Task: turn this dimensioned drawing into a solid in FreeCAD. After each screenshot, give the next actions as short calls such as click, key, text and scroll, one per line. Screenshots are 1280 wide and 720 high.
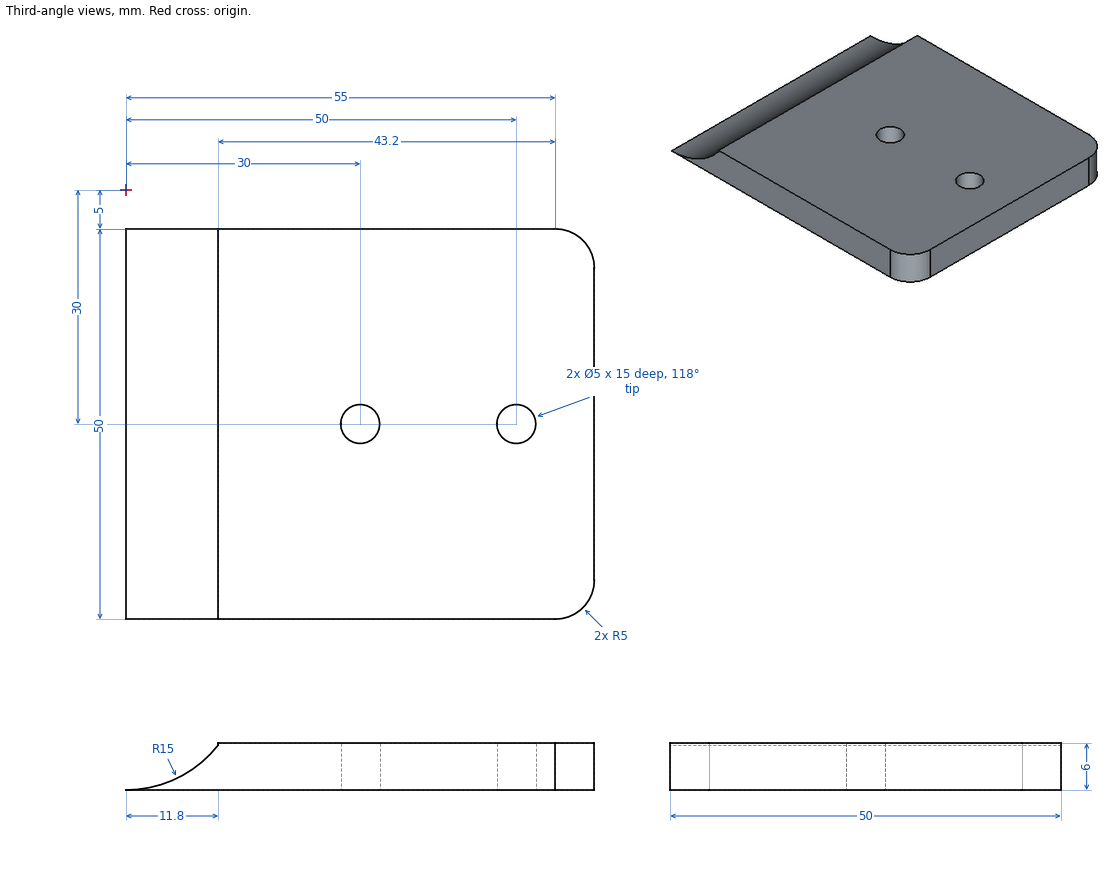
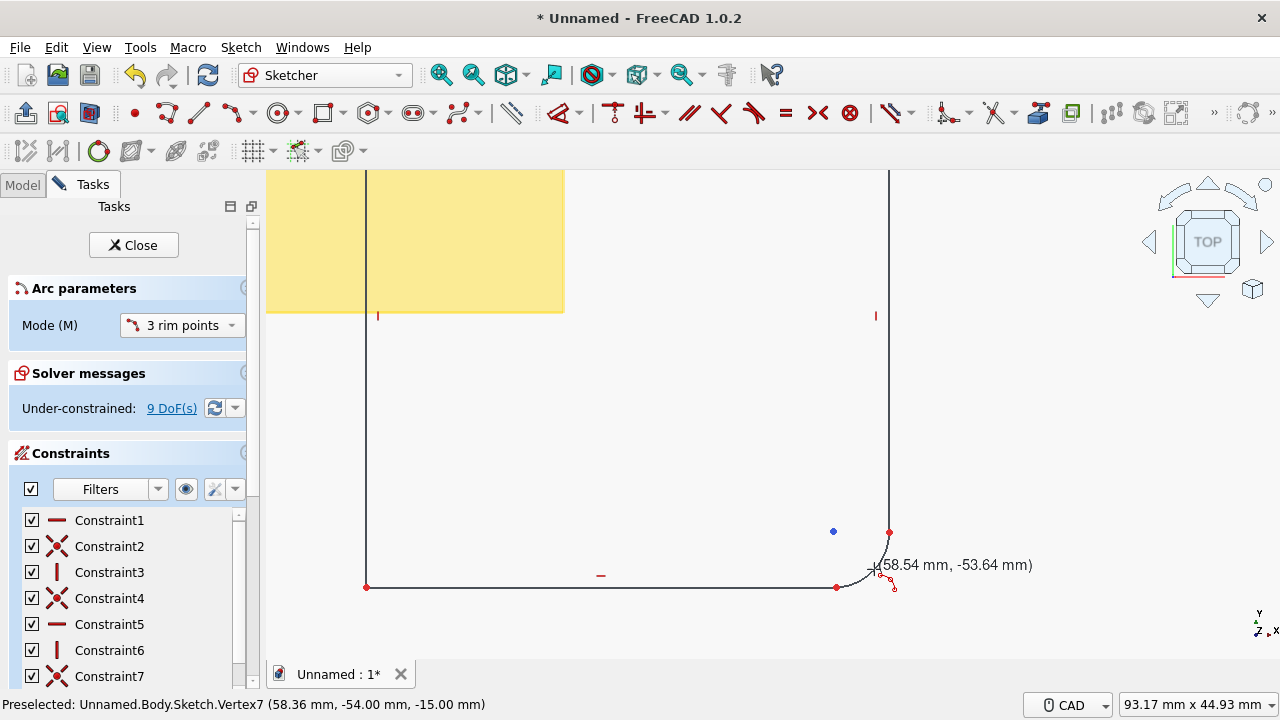
scroll(876, 571, down, 3)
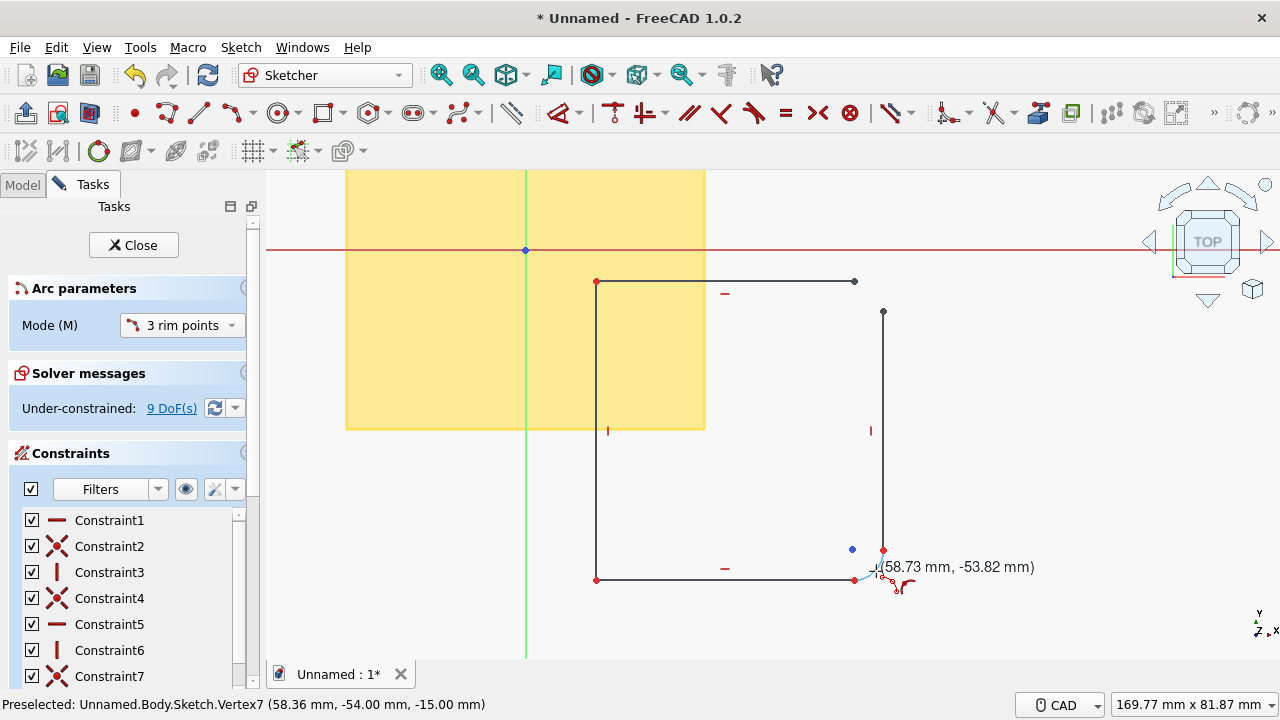
click(883, 311)
click(854, 281)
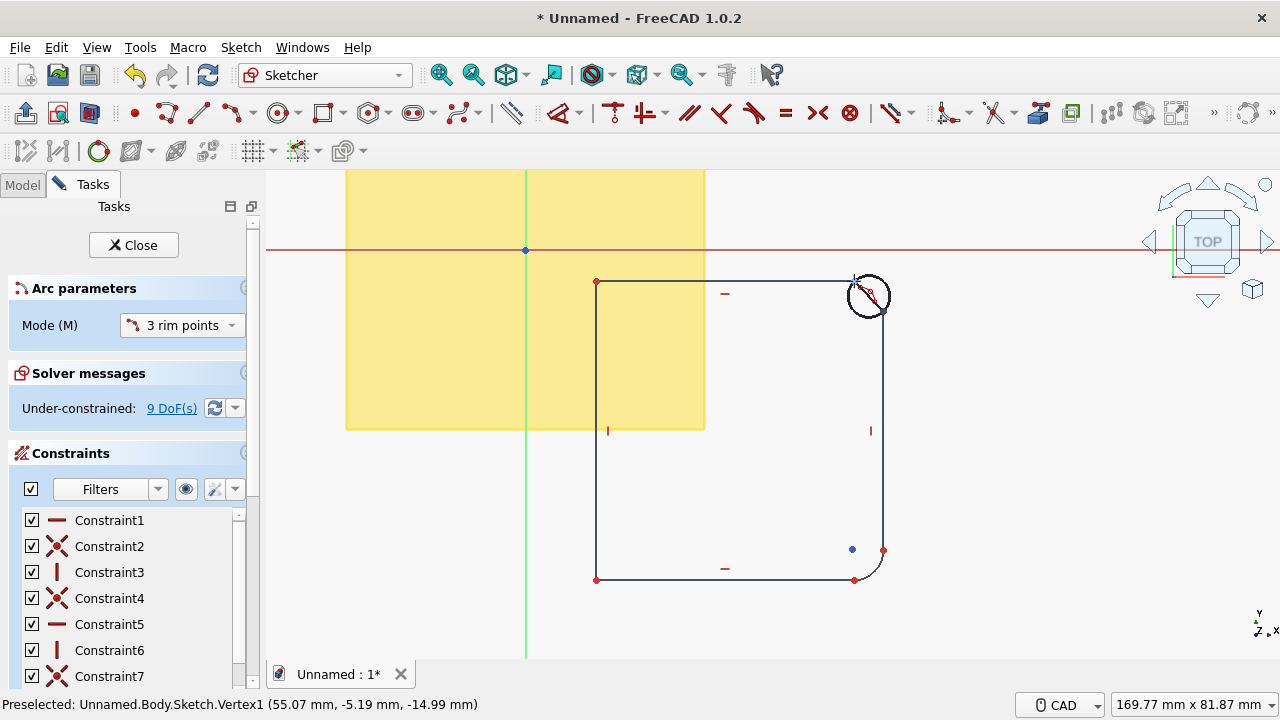
scroll(875, 289, up, 3)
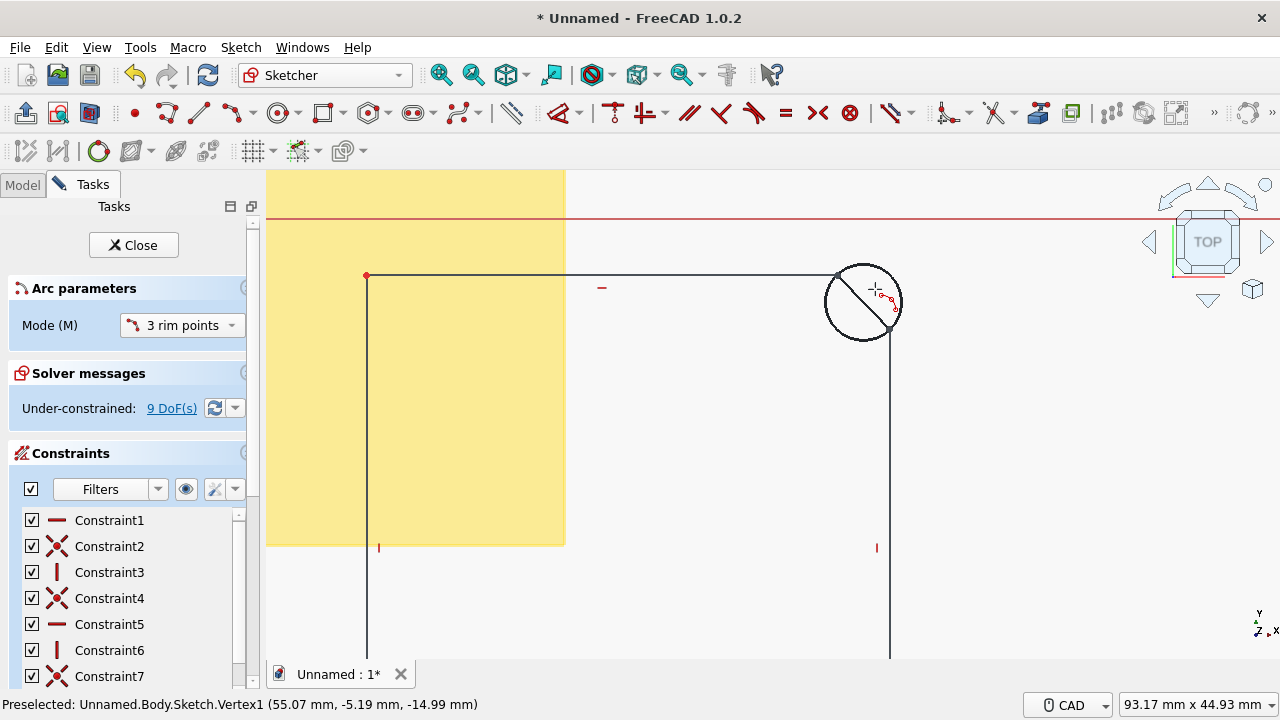
click(875, 289)
key(Escape)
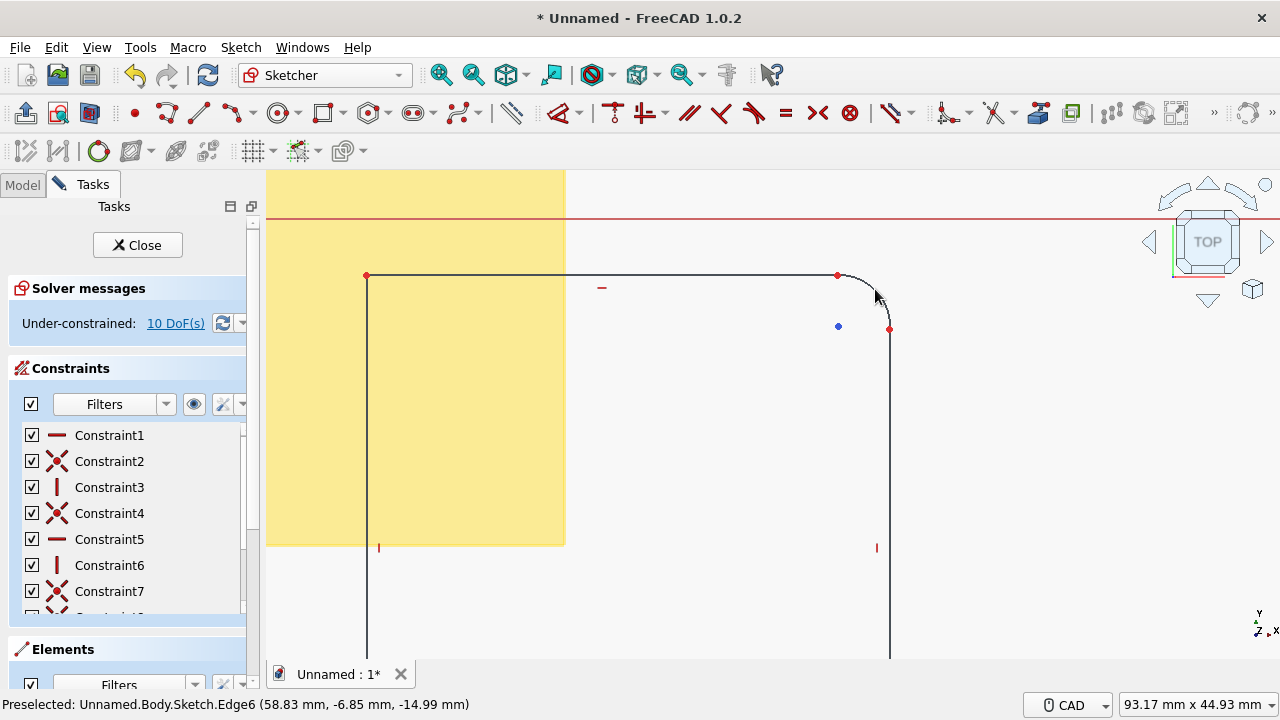
click(696, 275)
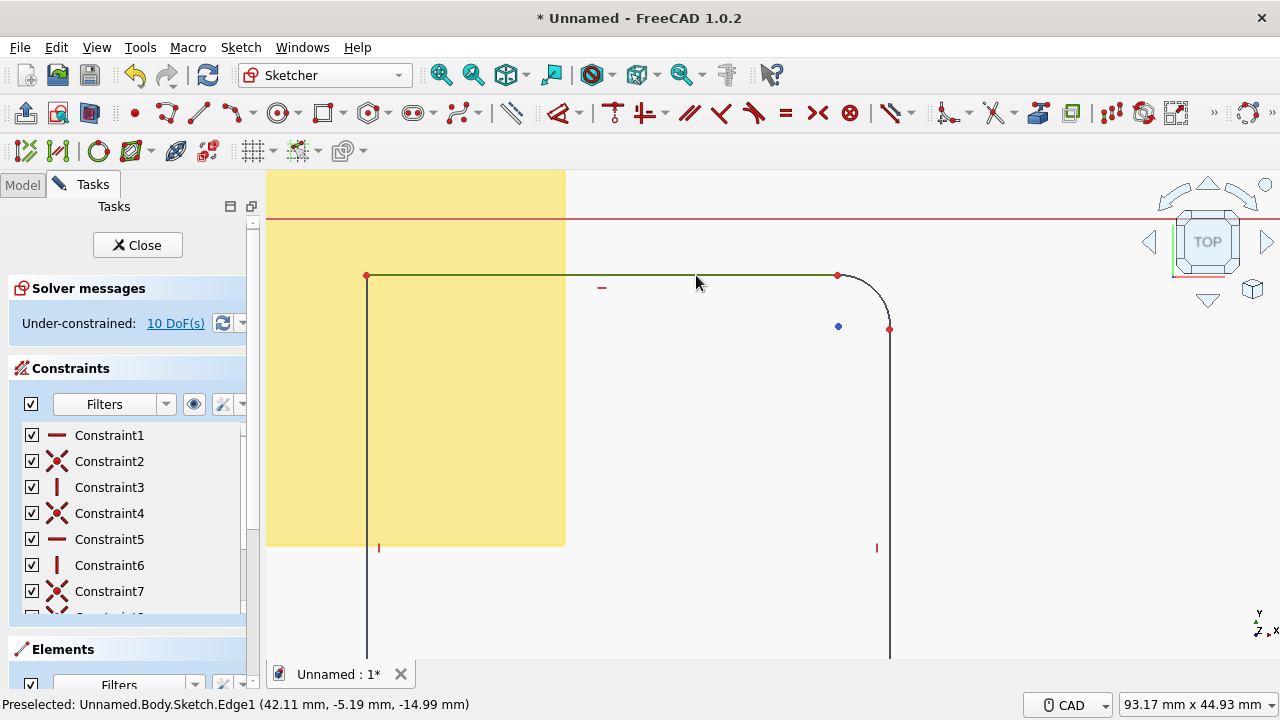
click(885, 305)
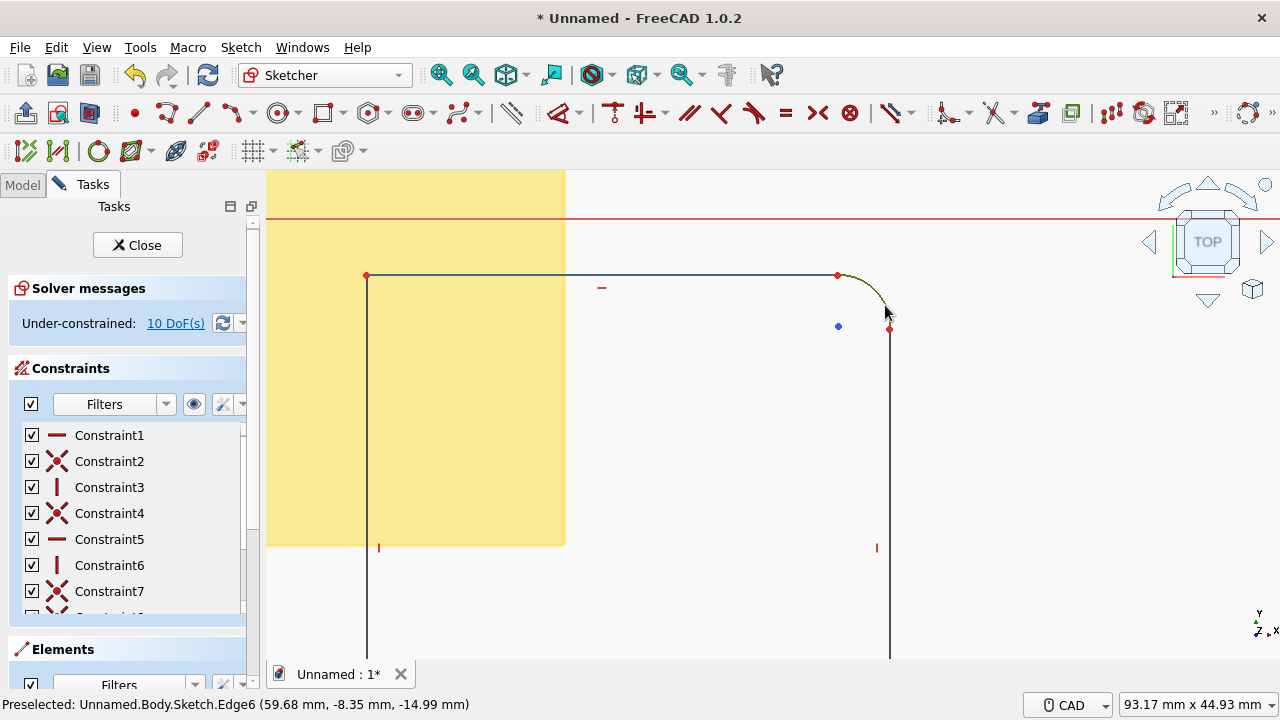
click(754, 114)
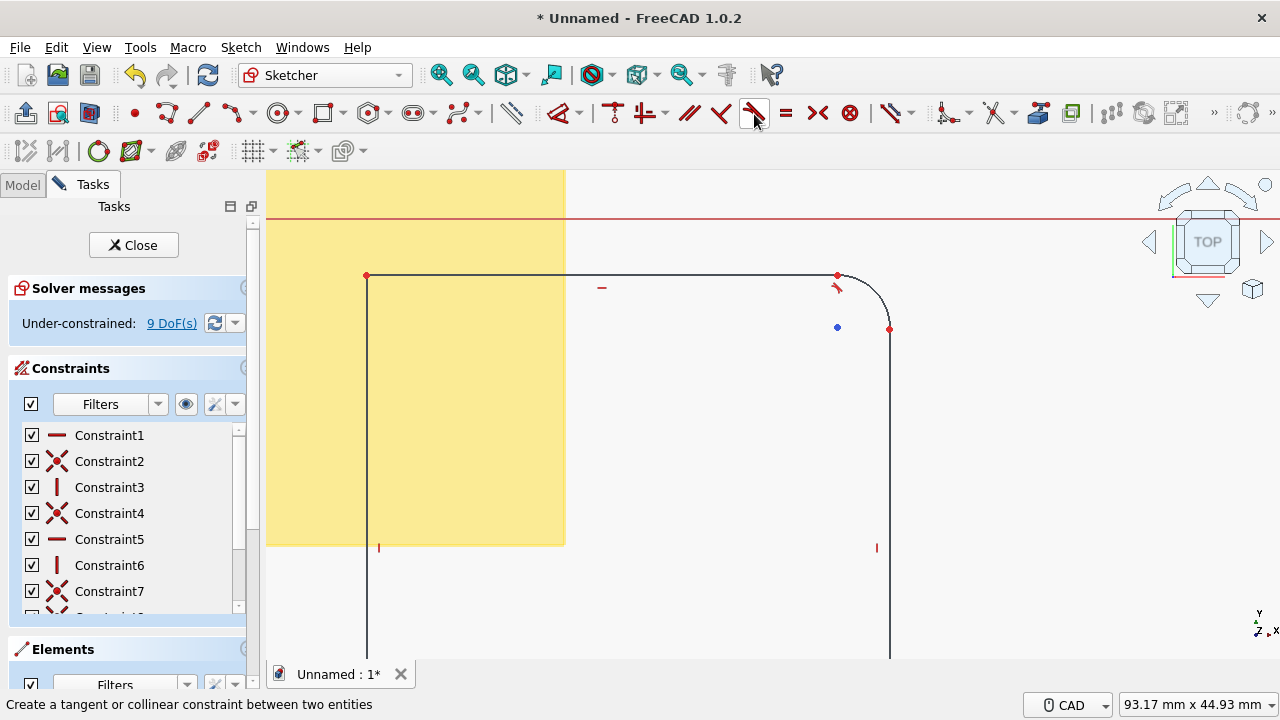
scroll(875, 289, down, 3)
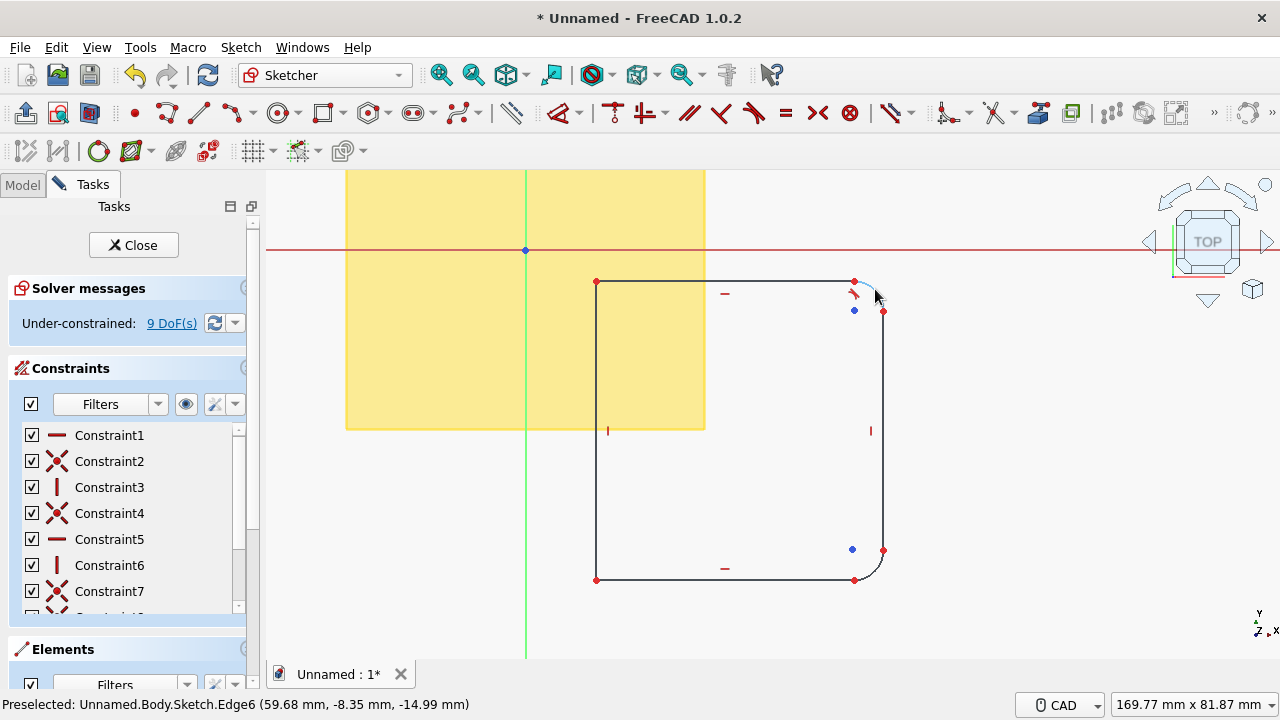
click(674, 580)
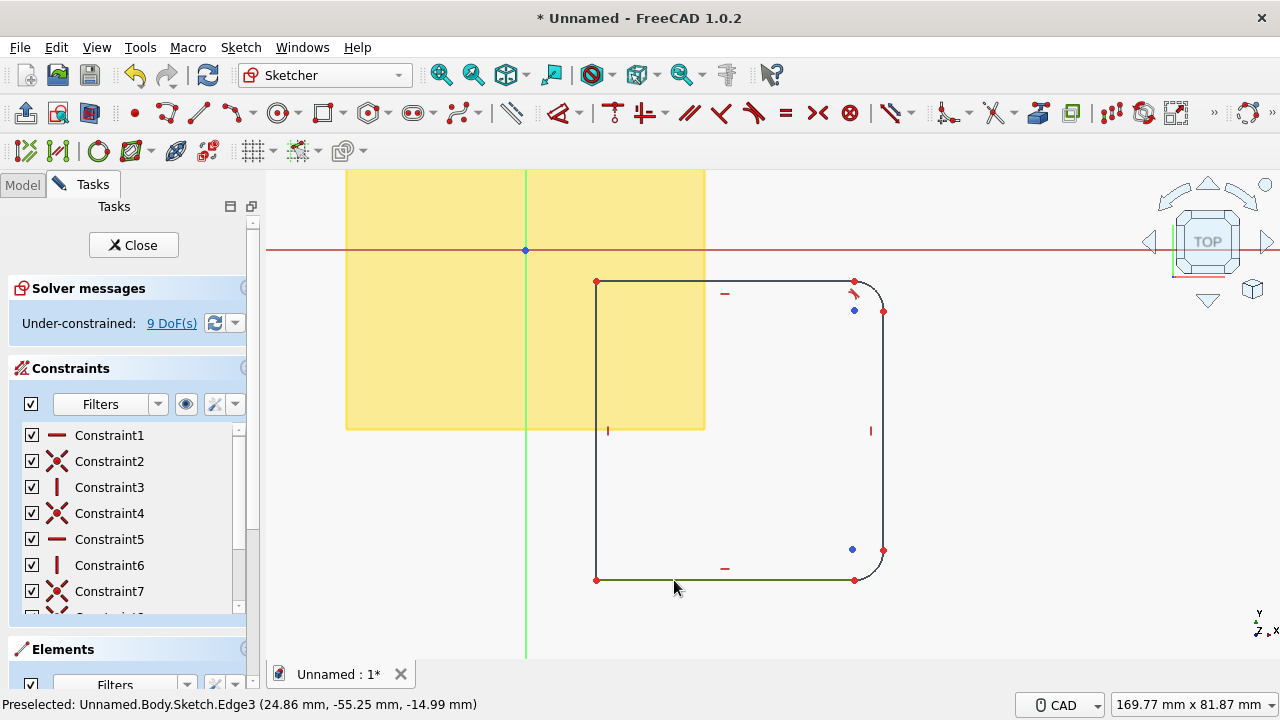
click(868, 577)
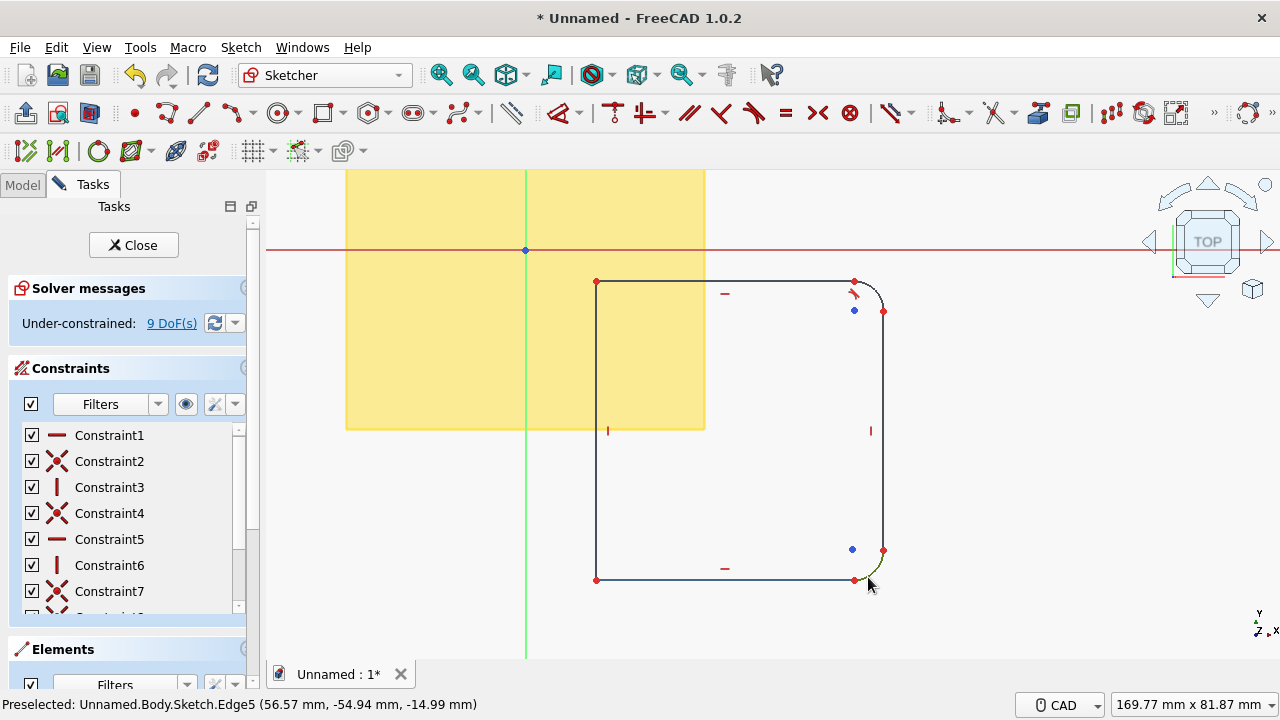
click(754, 114)